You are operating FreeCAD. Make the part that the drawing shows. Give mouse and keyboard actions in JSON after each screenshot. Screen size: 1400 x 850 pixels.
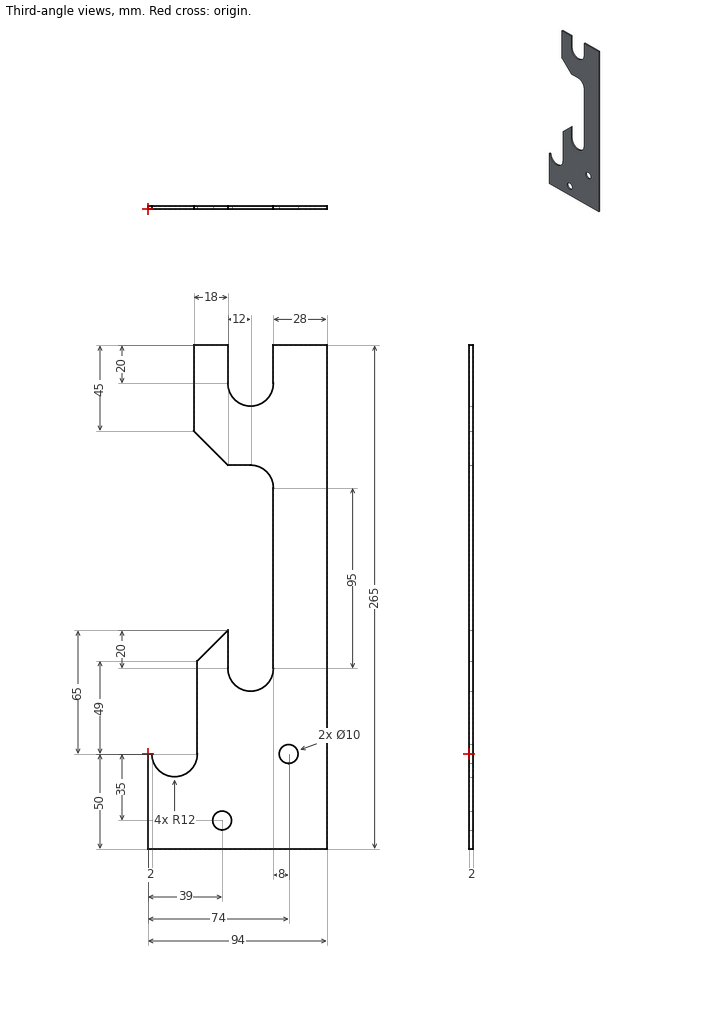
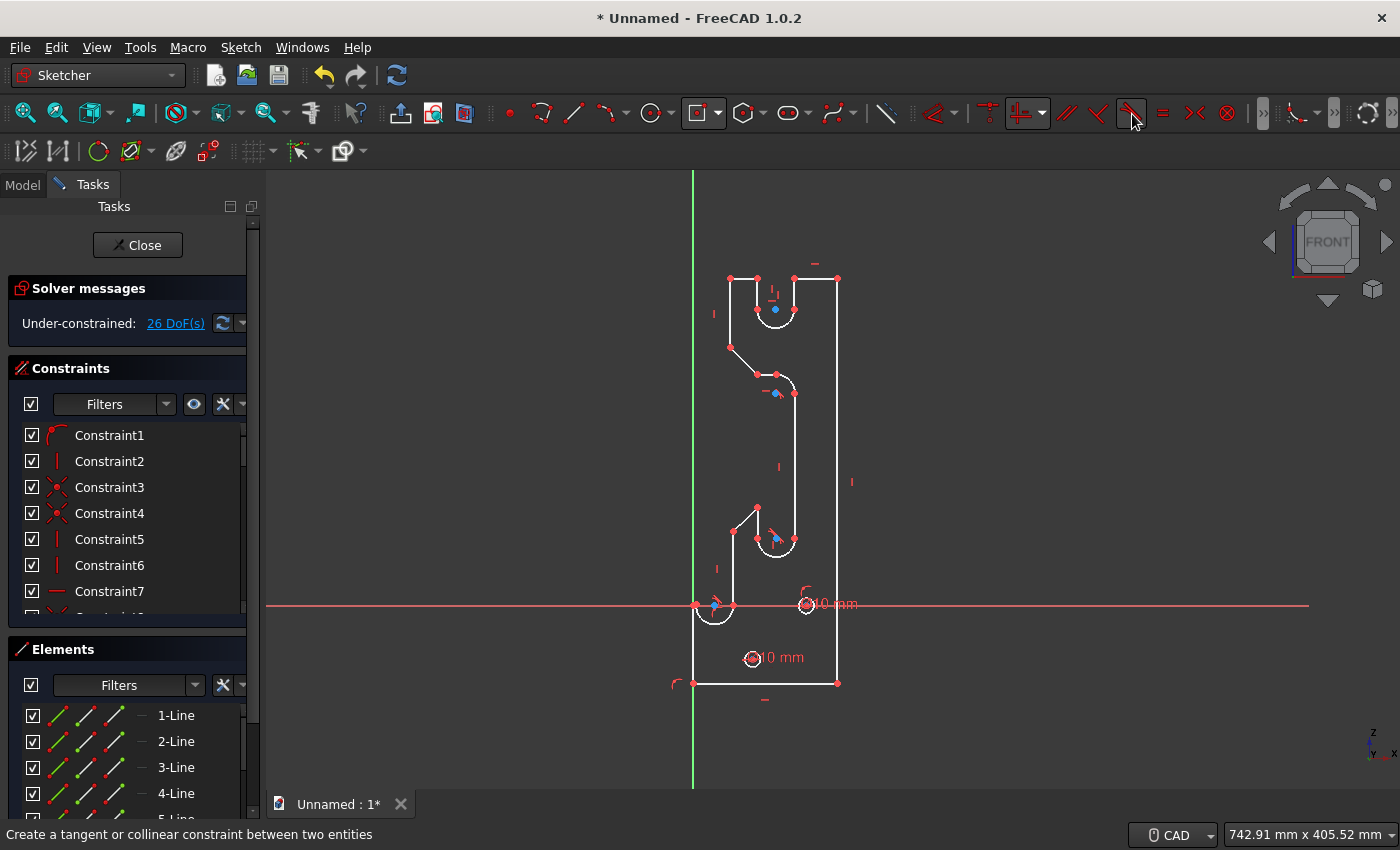
{"action": "scroll", "coordinate": [767, 375], "scroll_direction": "up", "scroll_amount": 2}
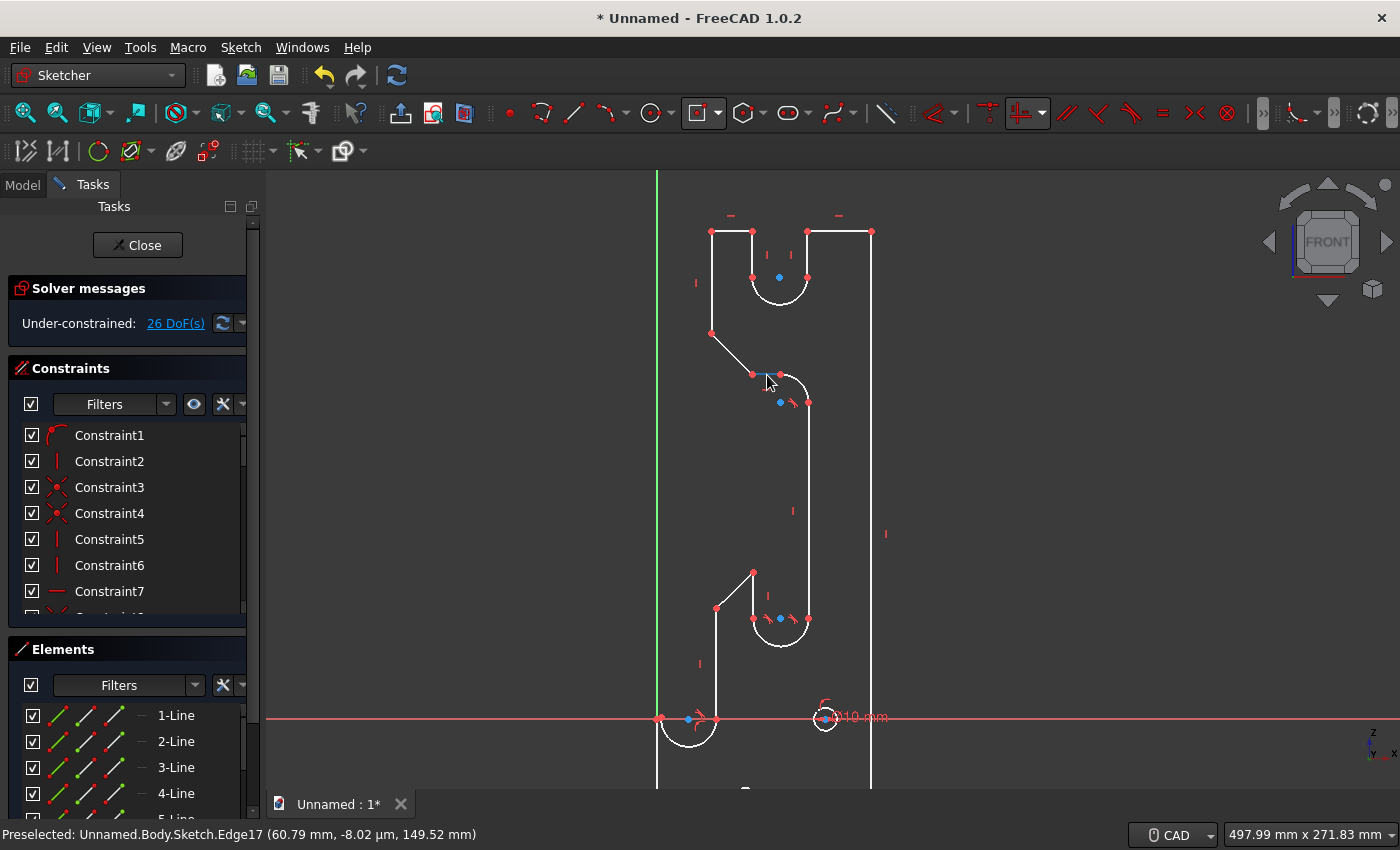
{"action": "left_click", "coordinate": [766, 374]}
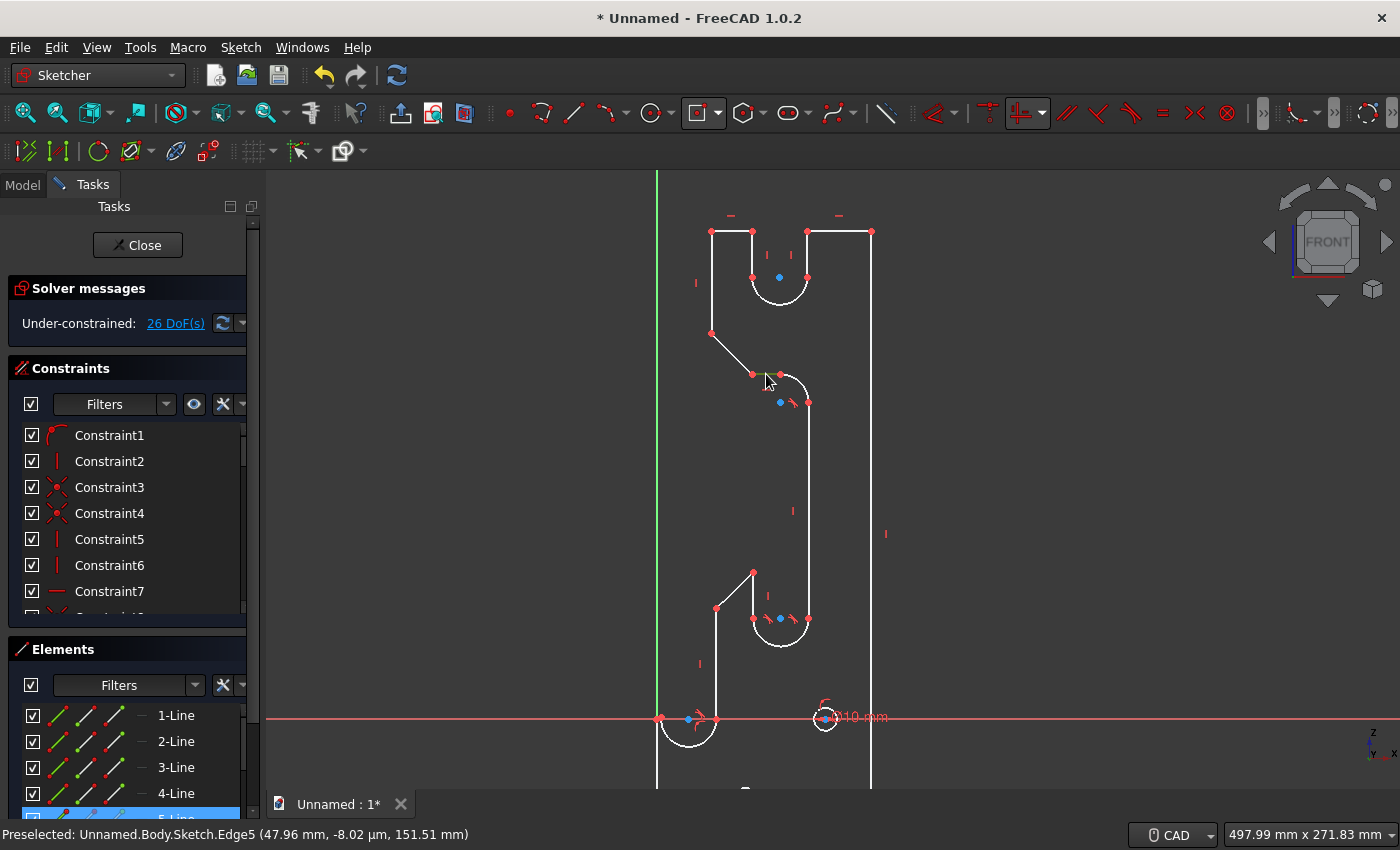
{"action": "left_click", "coordinate": [805, 390]}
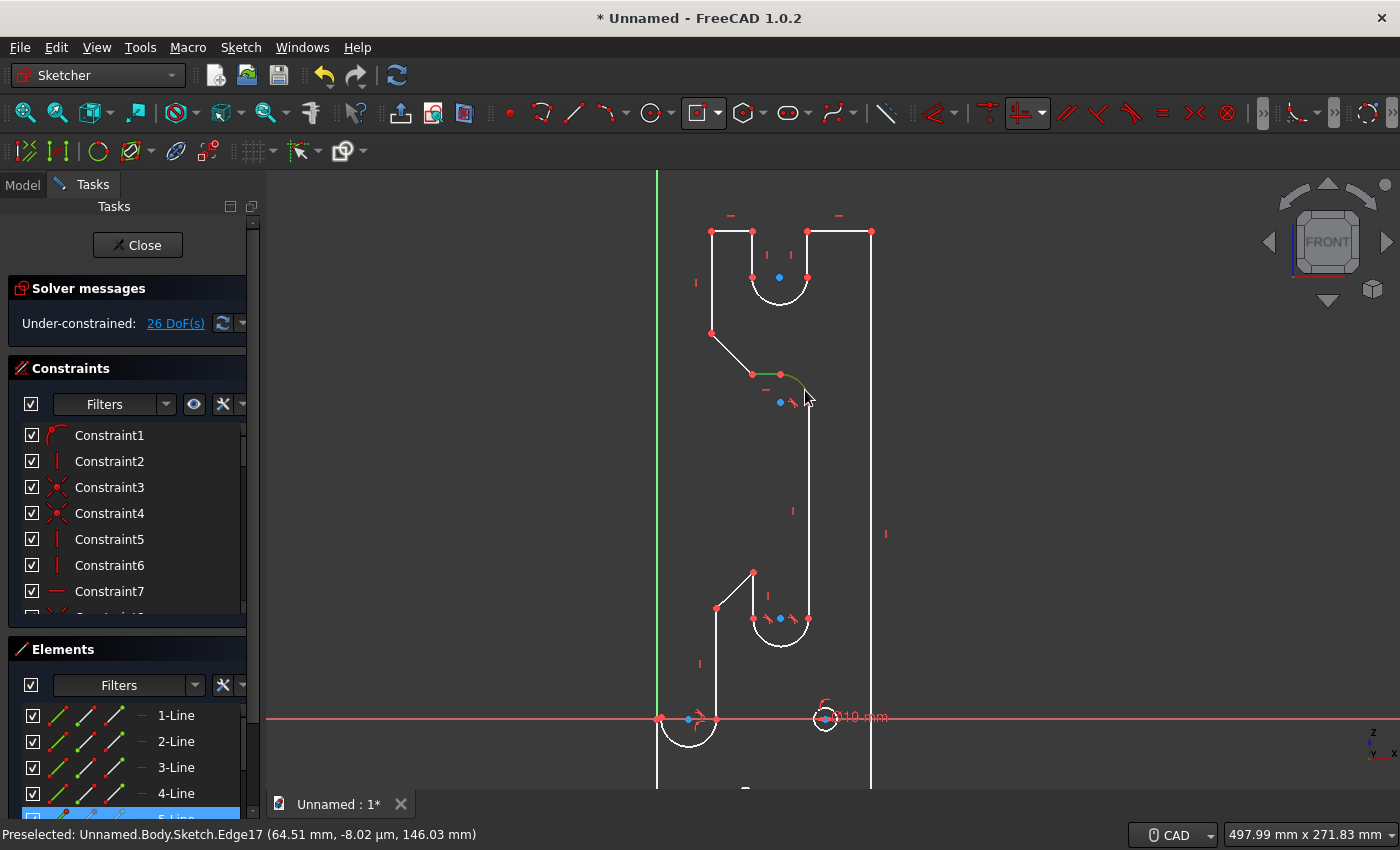
{"action": "key", "text": "t"}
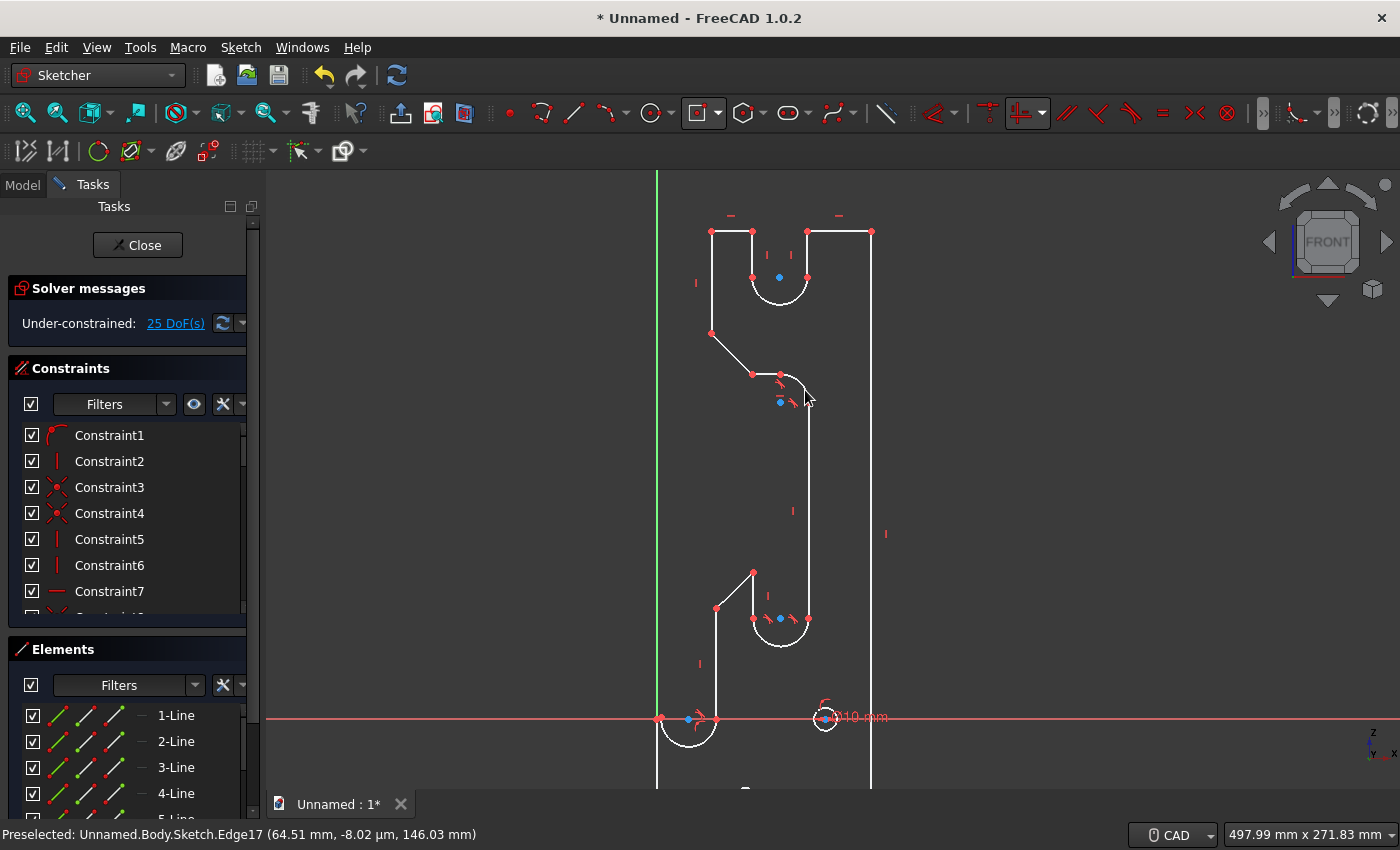
{"action": "left_click", "coordinate": [752, 245]}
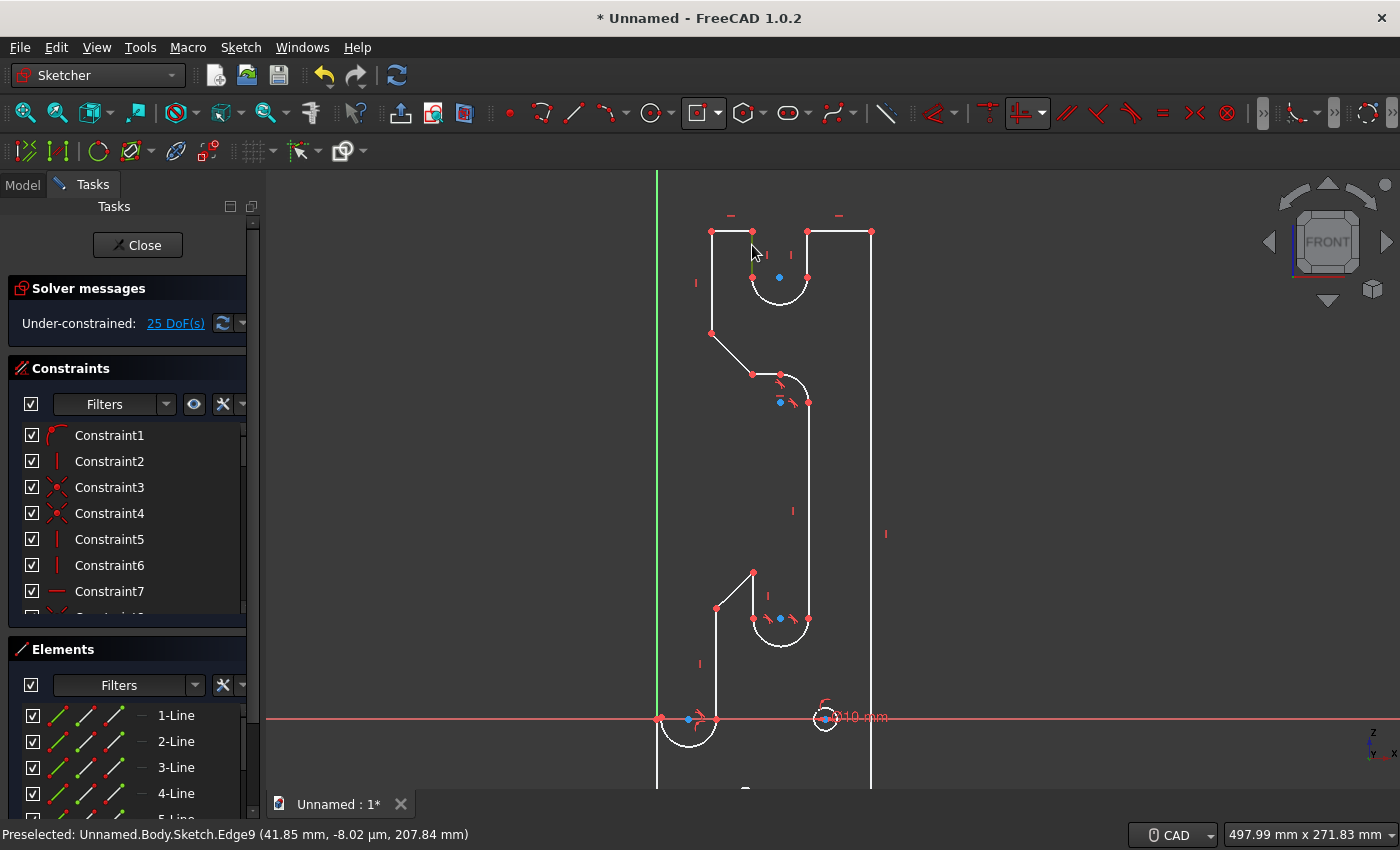
{"action": "left_click", "coordinate": [764, 299]}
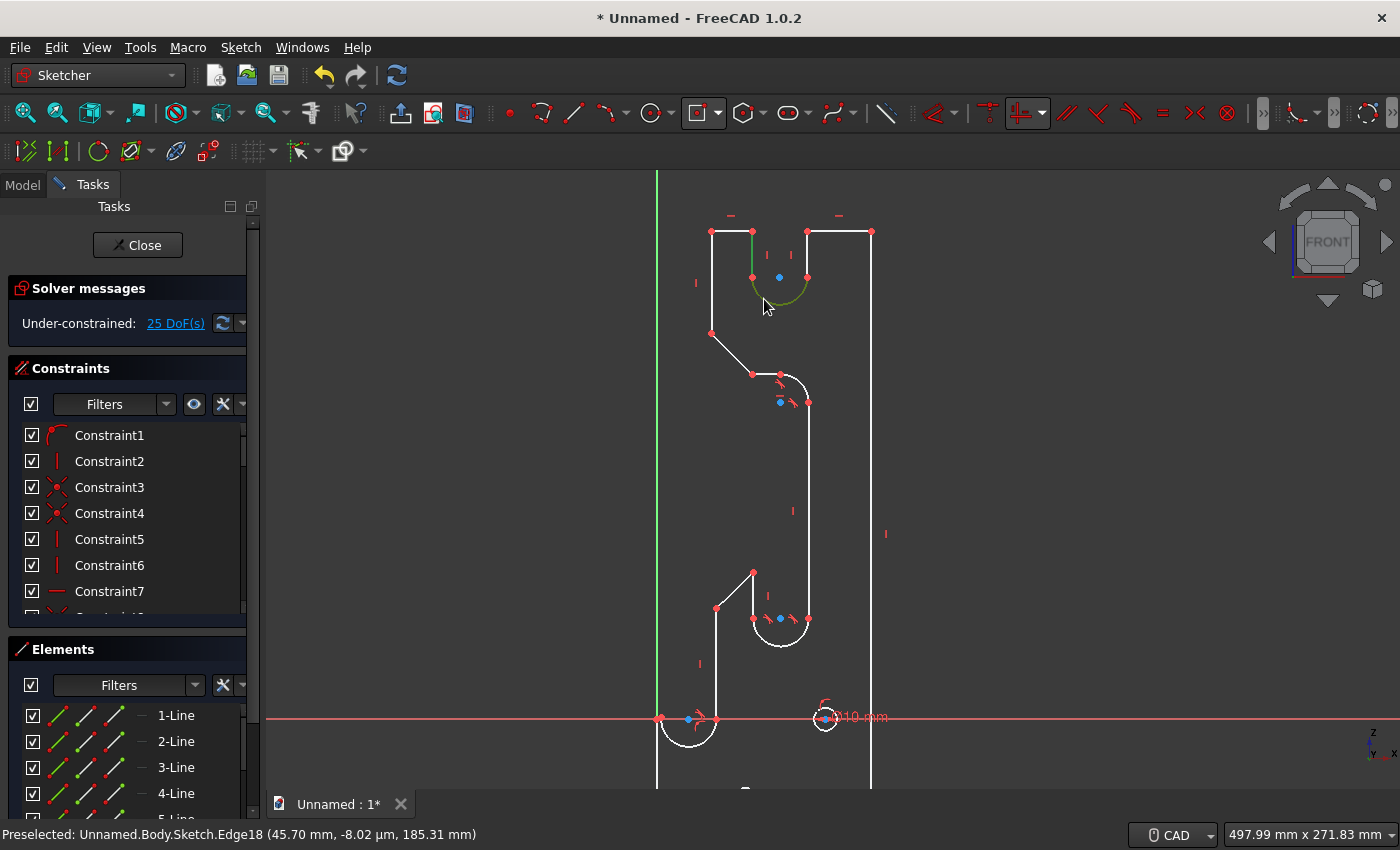
{"action": "left_click", "coordinate": [1132, 114]}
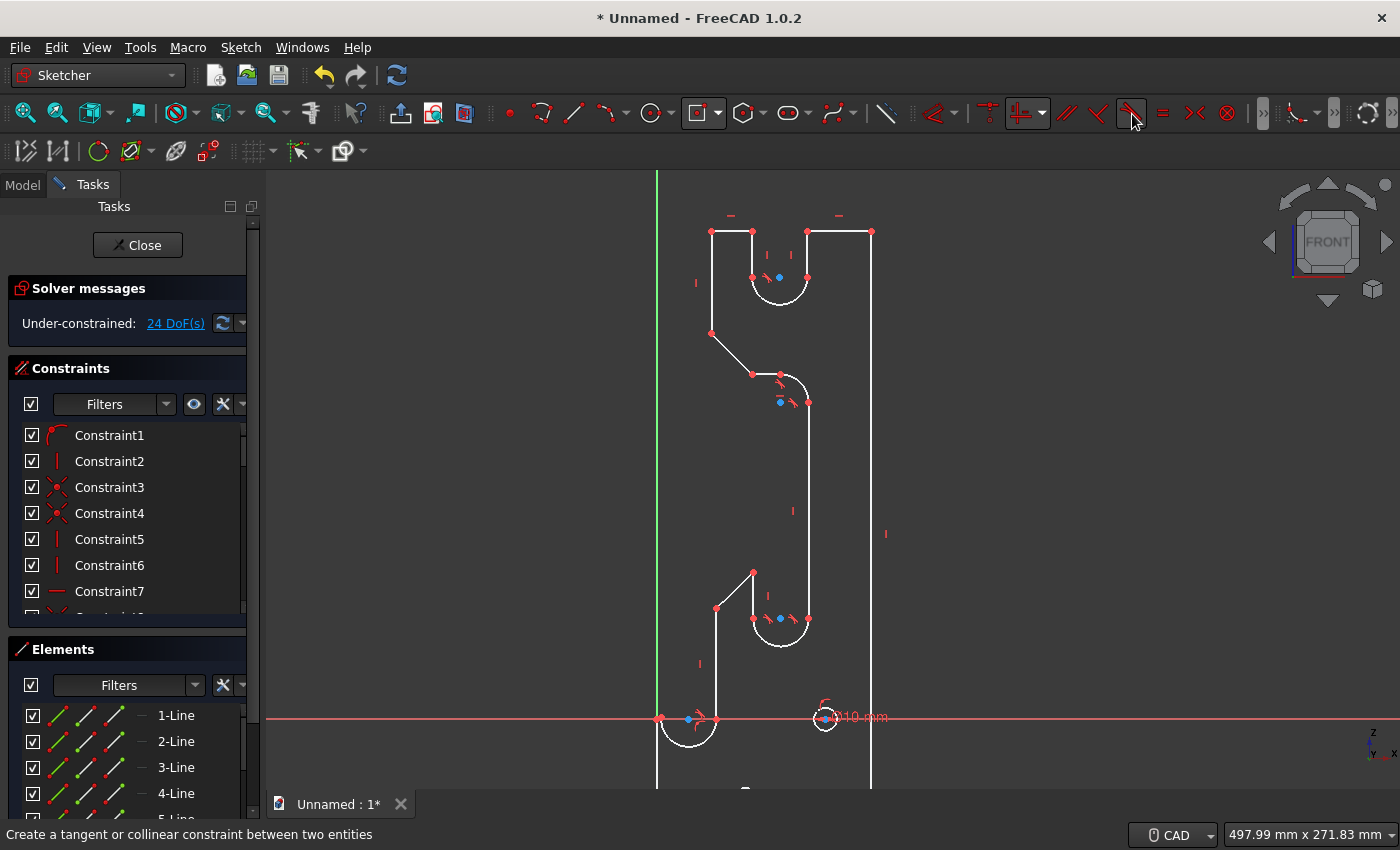
{"action": "left_click", "coordinate": [807, 263]}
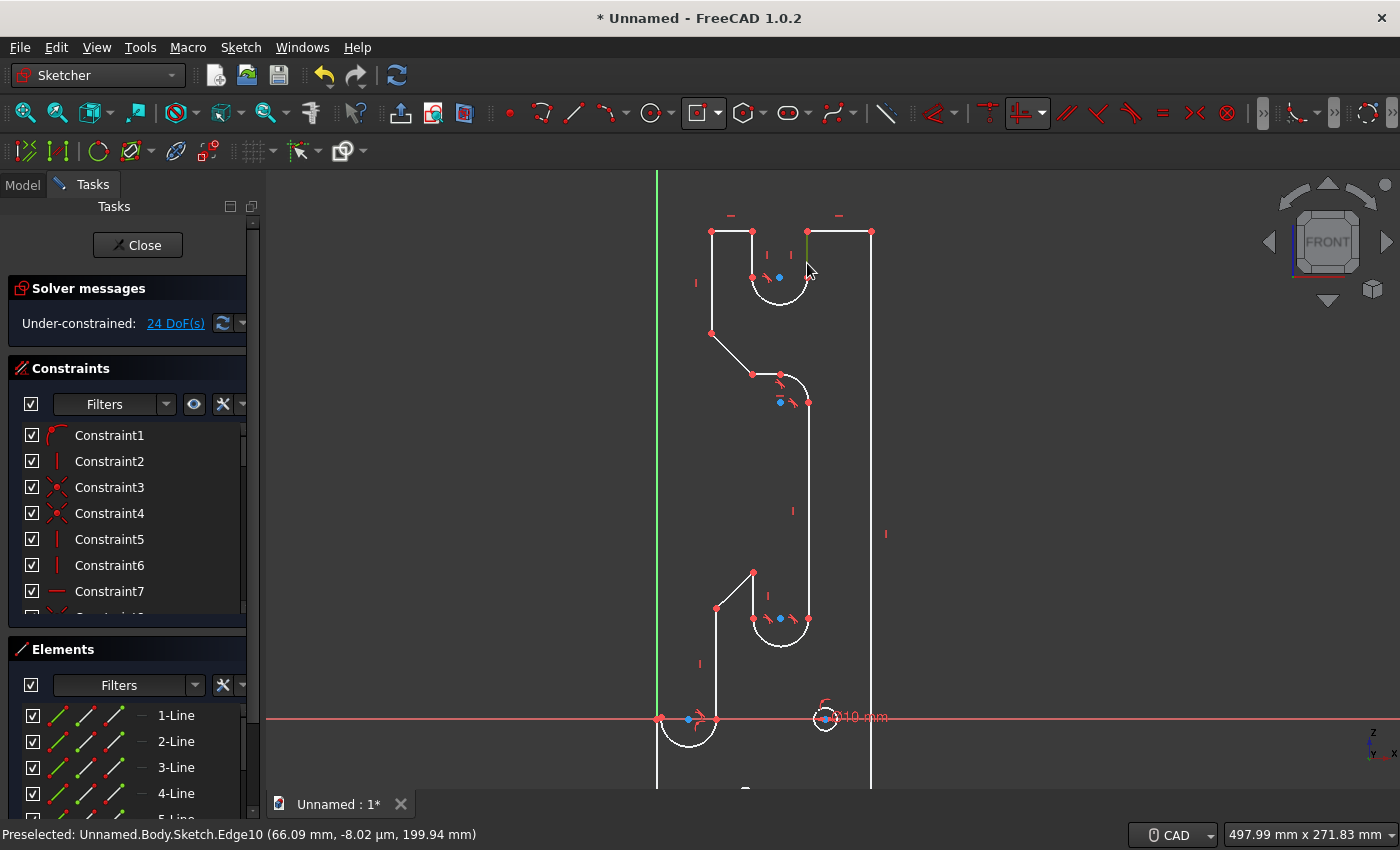
{"action": "left_click", "coordinate": [763, 299]}